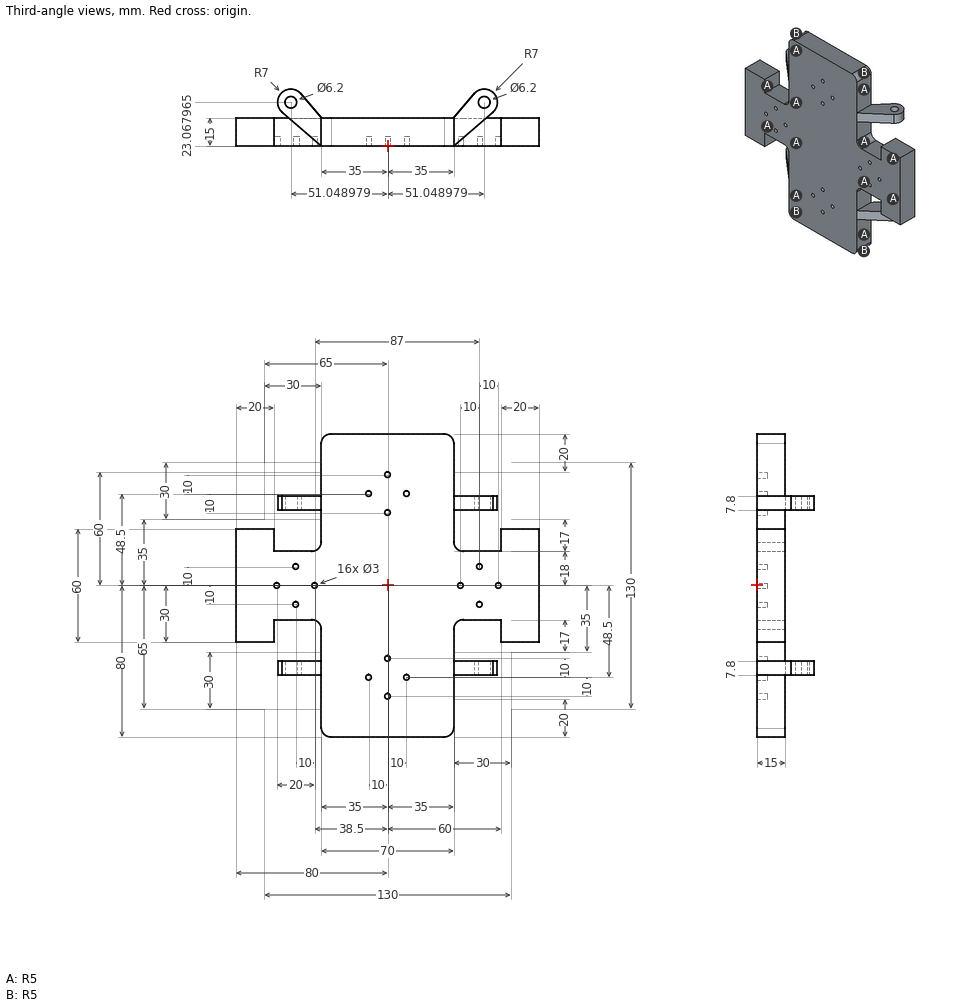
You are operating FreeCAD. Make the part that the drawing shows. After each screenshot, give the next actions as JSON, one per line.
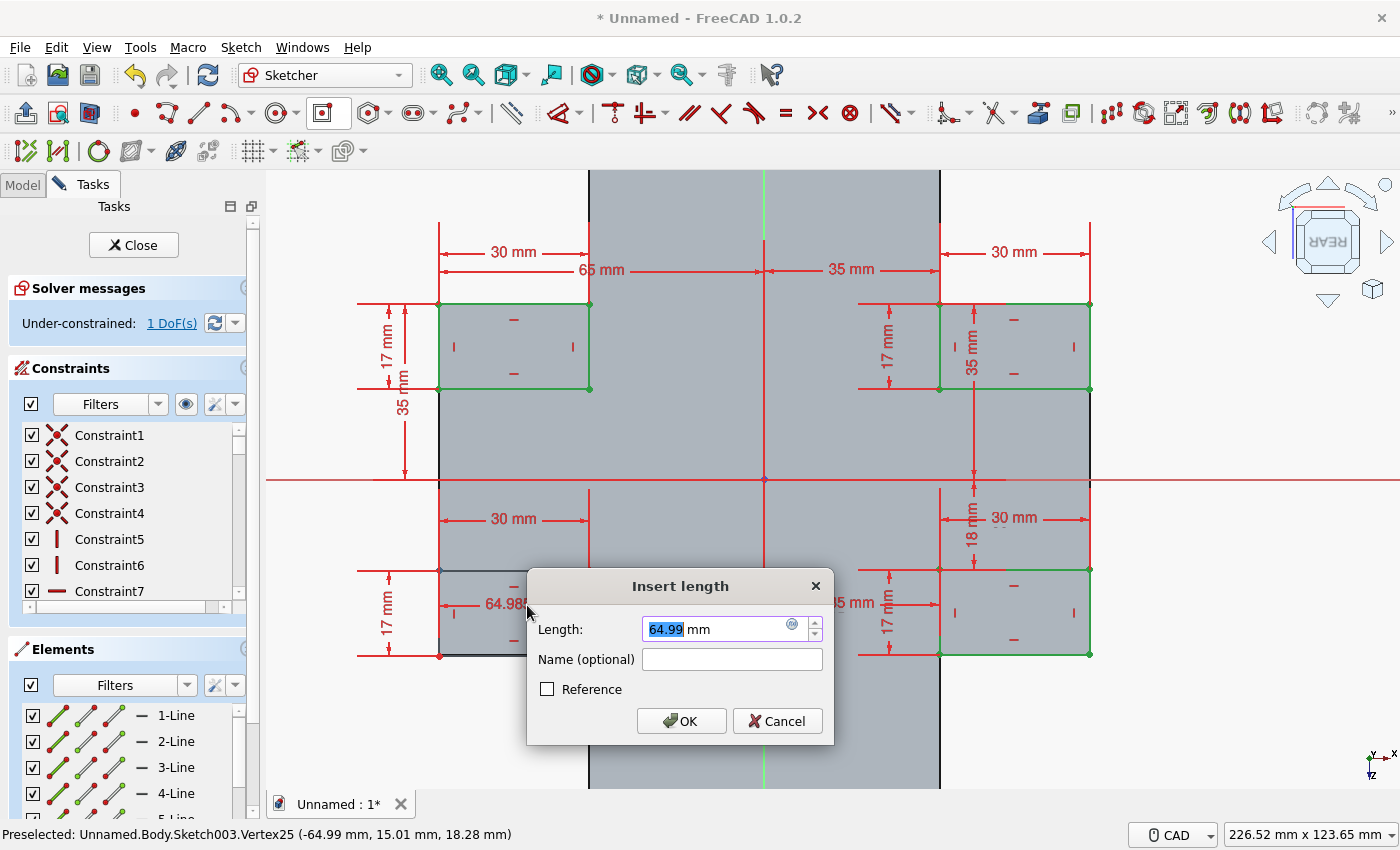
{"action": "type", "text": "65"}
{"action": "key", "text": "Return"}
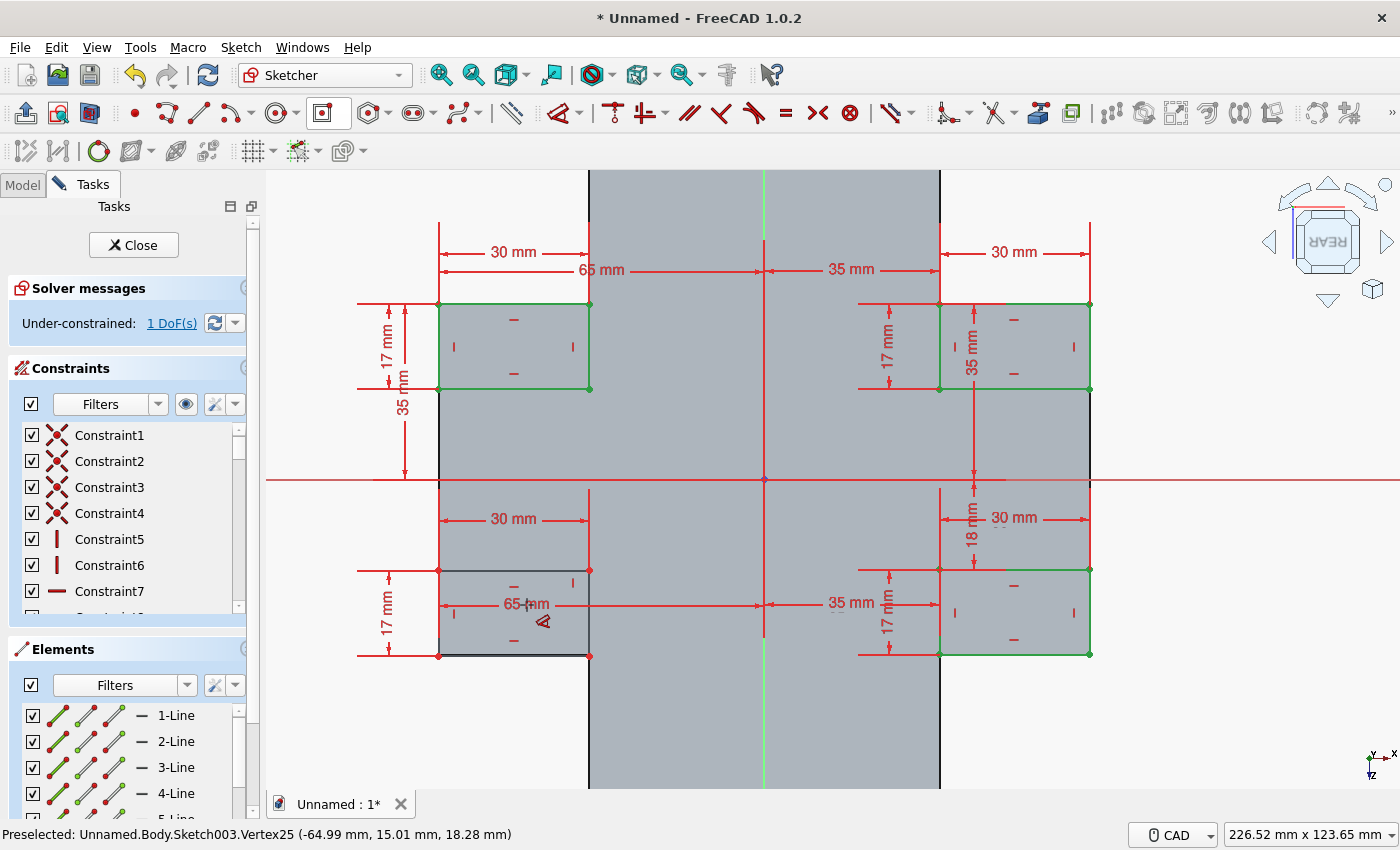
{"action": "left_click", "coordinate": [439, 571]}
{"action": "left_click", "coordinate": [405, 525]}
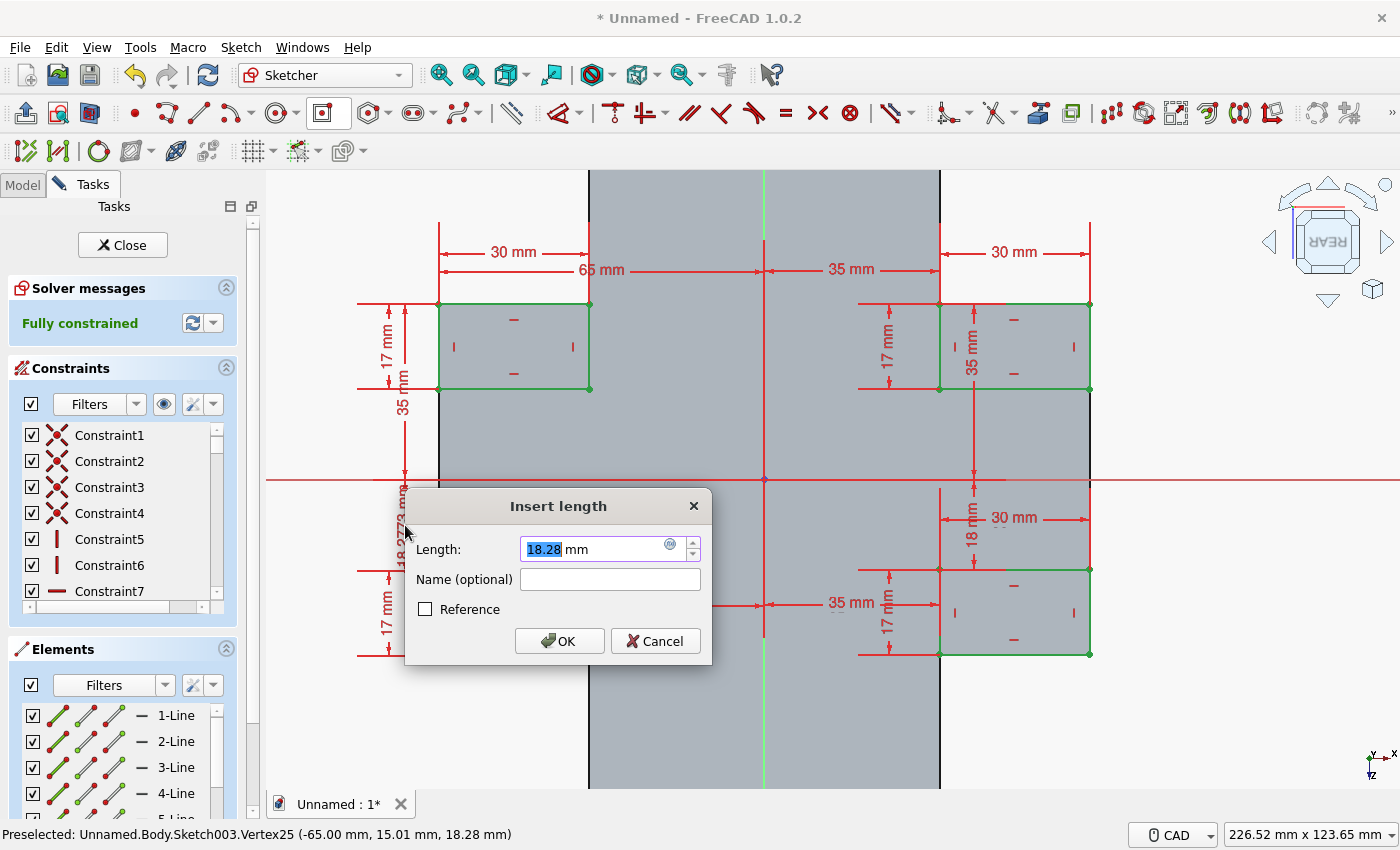
{"action": "type", "text": "18"}
{"action": "key", "text": "Return"}
{"action": "key", "text": "Escape"}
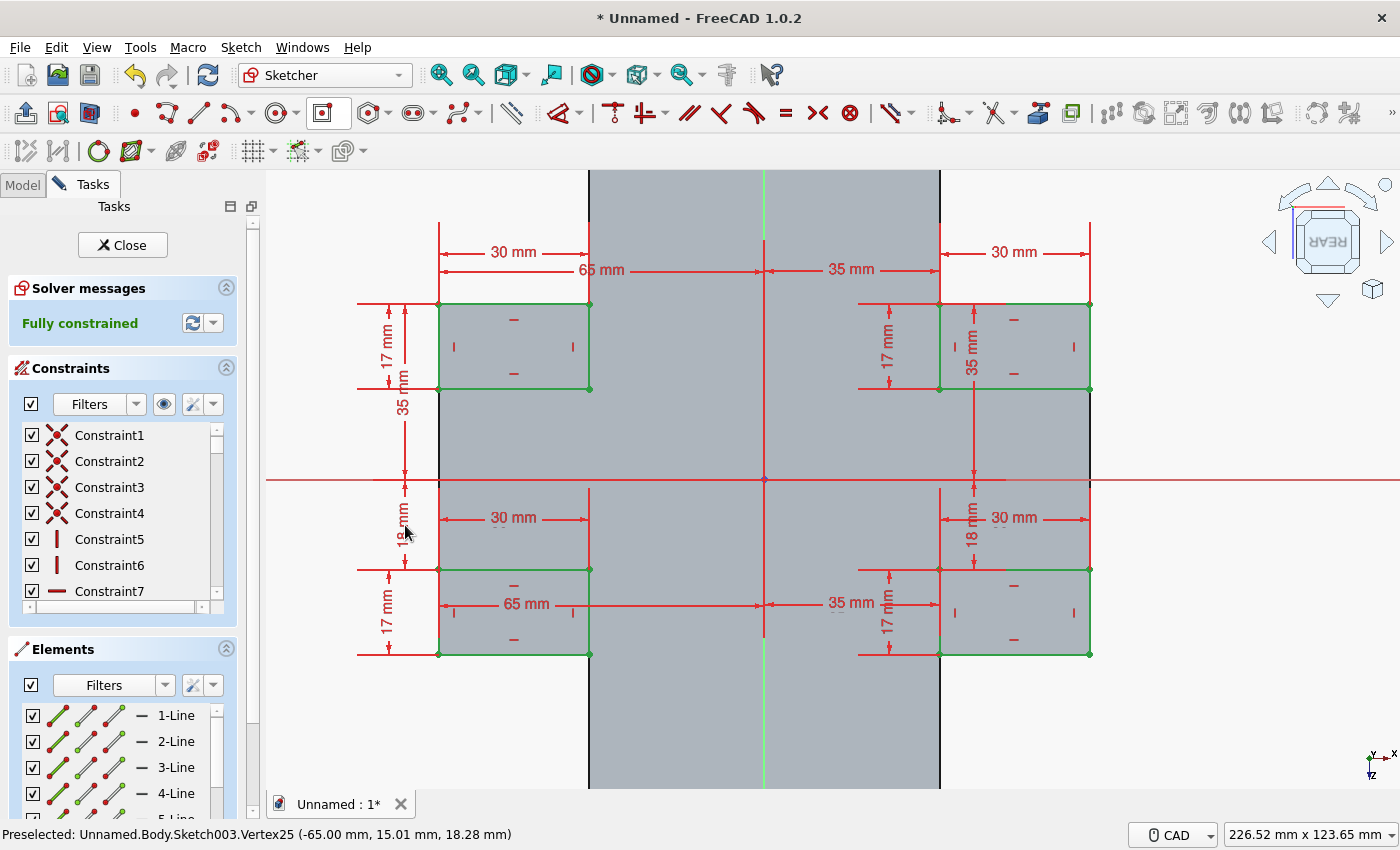
{"action": "left_click", "coordinate": [123, 245]}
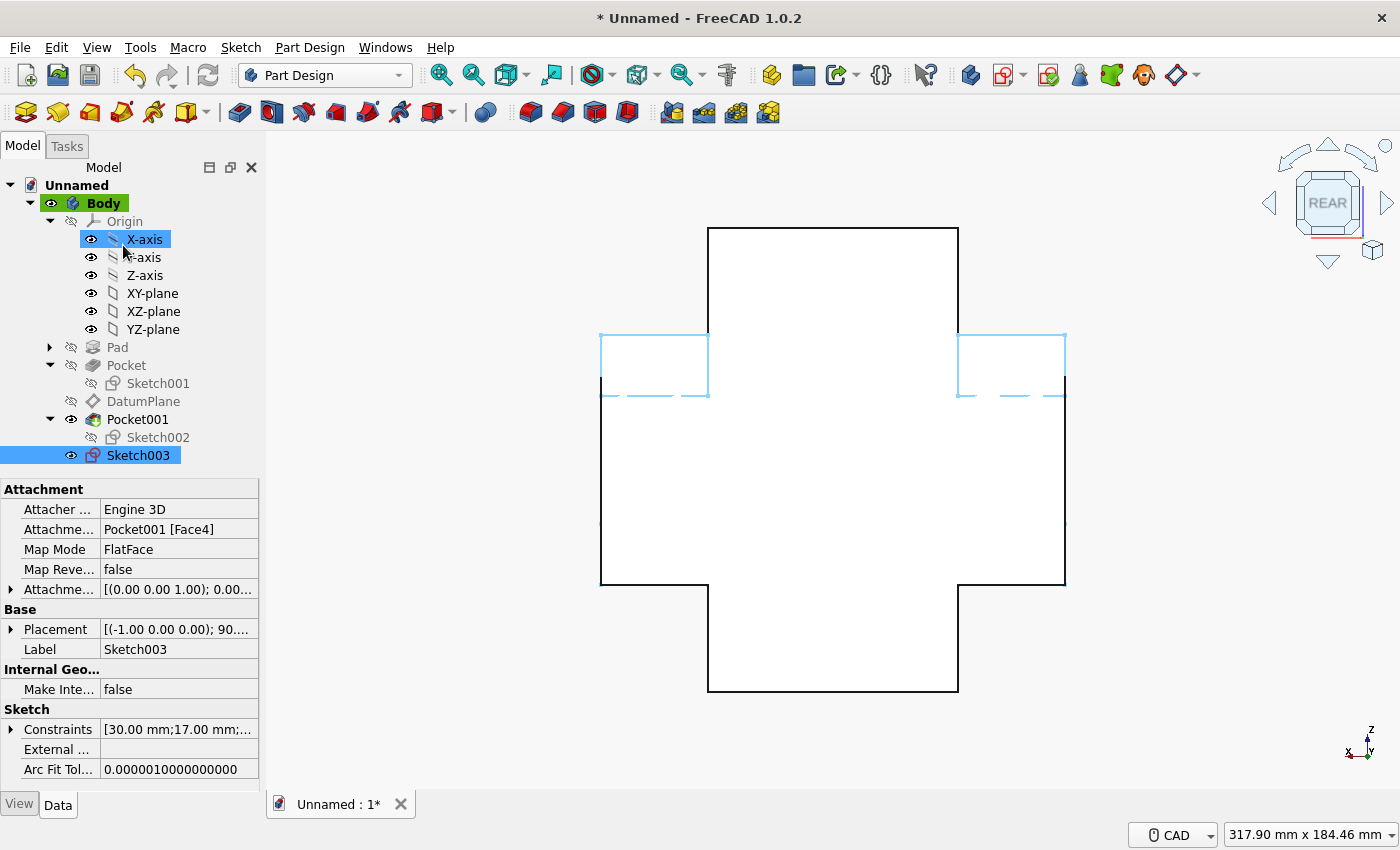
{"action": "left_click", "coordinate": [240, 112]}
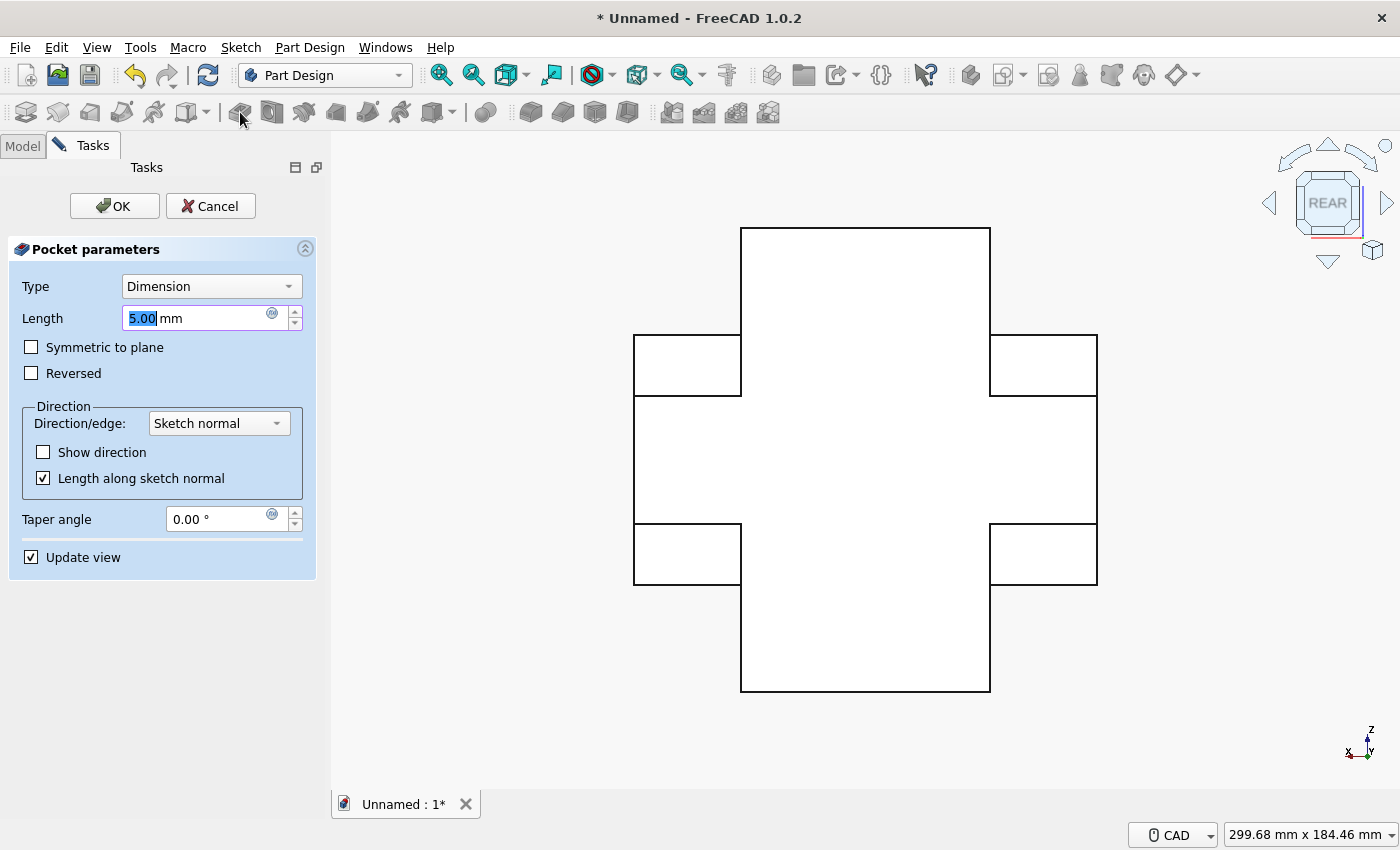
{"action": "left_click", "coordinate": [212, 286]}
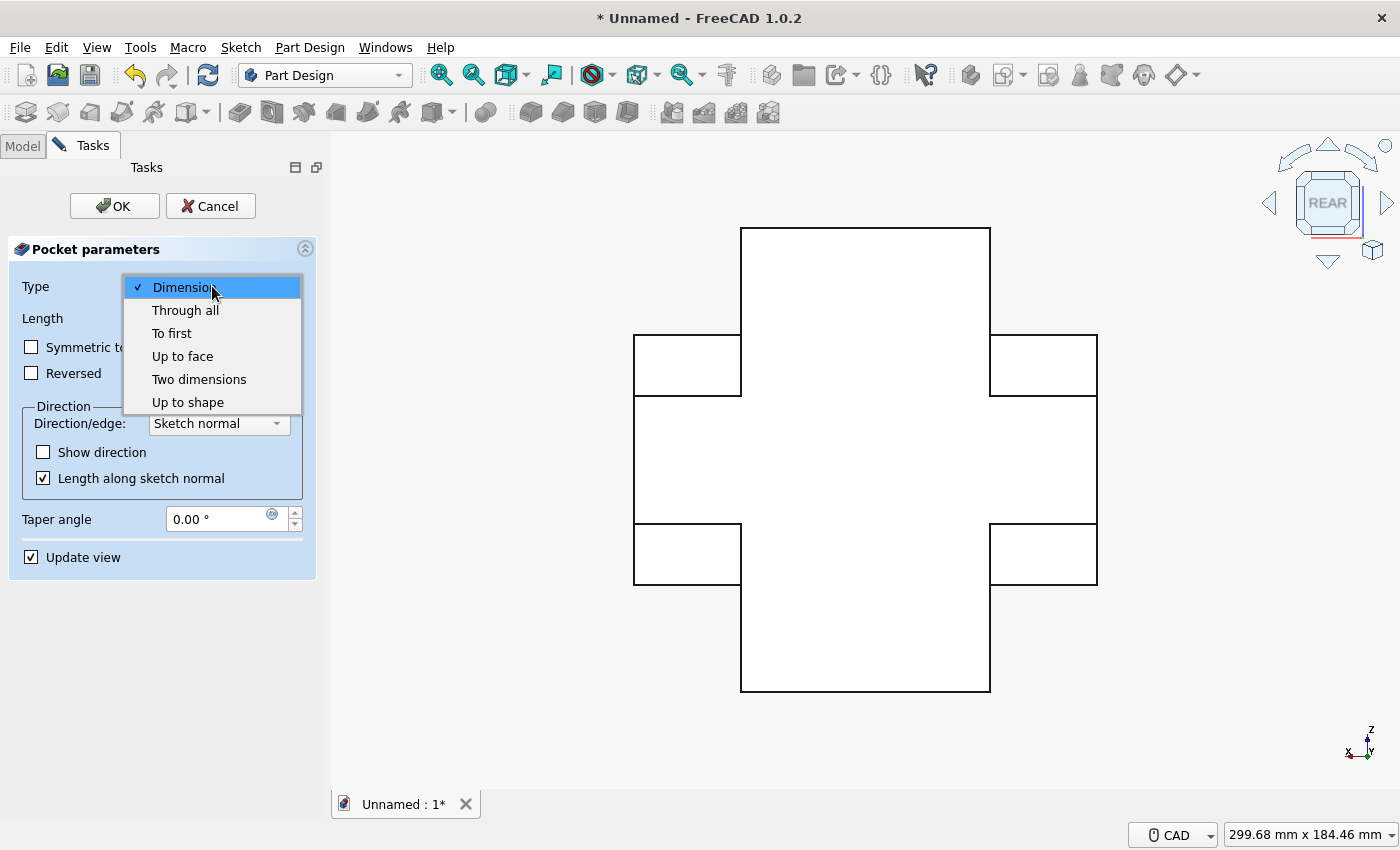
{"action": "left_click", "coordinate": [212, 310]}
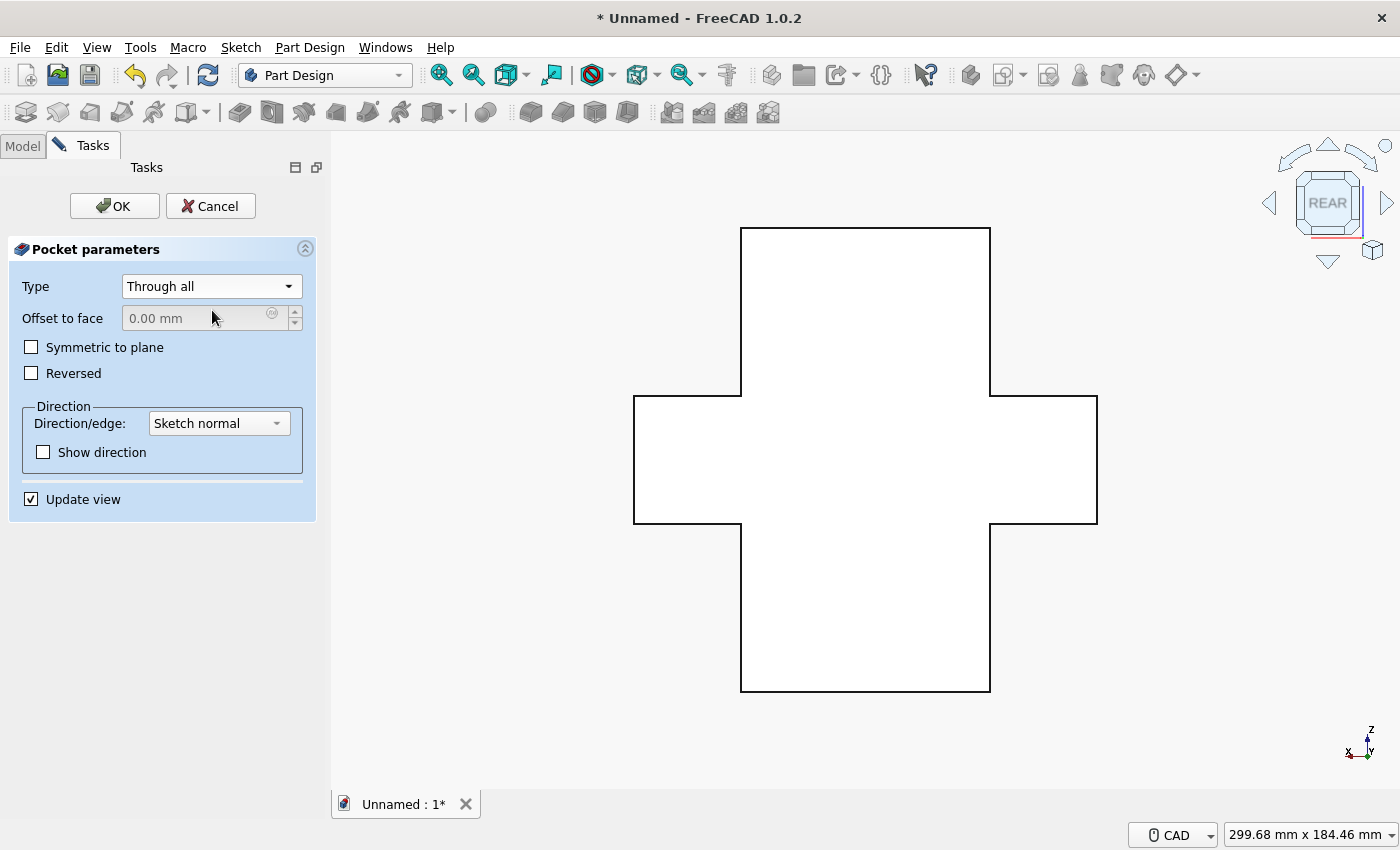
{"action": "left_click", "coordinate": [115, 206]}